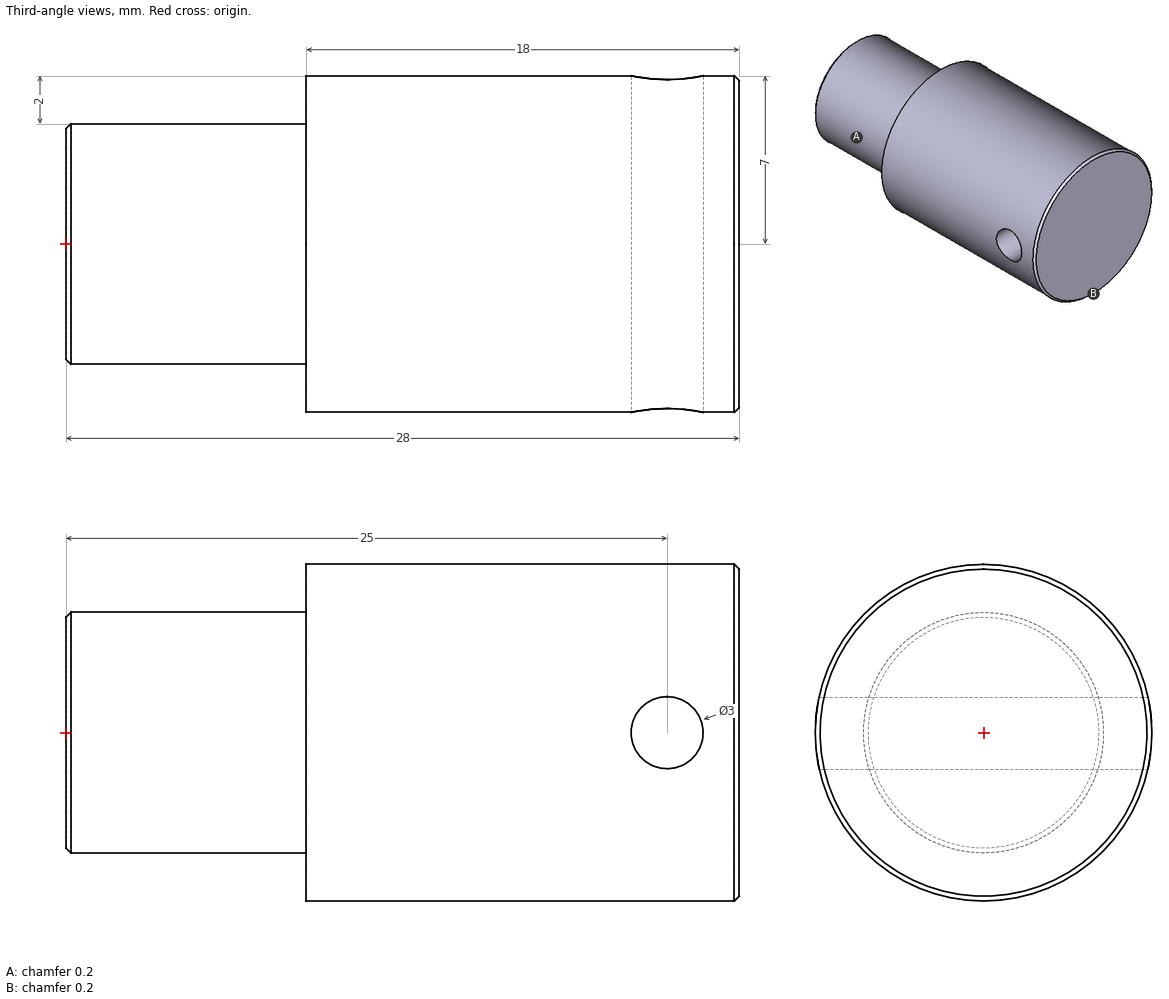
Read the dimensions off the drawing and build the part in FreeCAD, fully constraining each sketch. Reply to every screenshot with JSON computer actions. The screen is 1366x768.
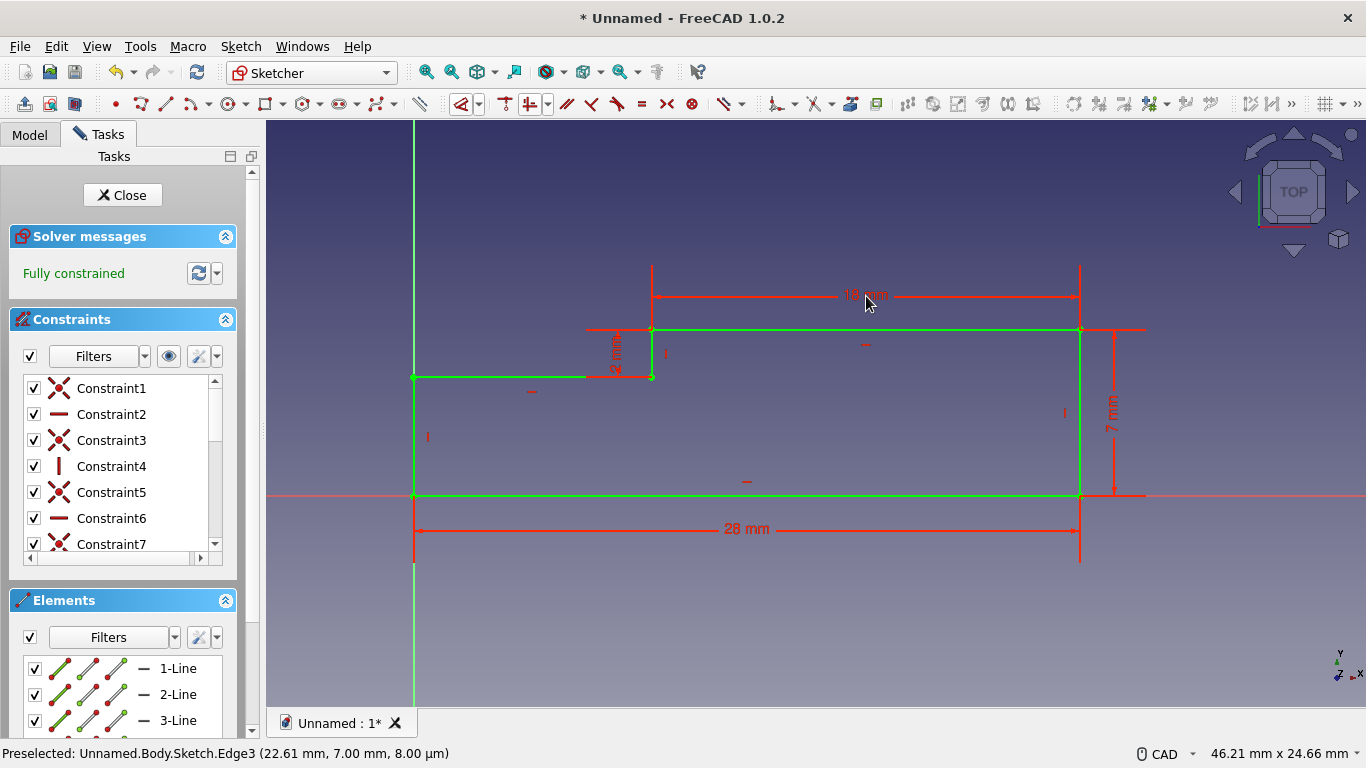
{"action": "left_click", "coordinate": [123, 195]}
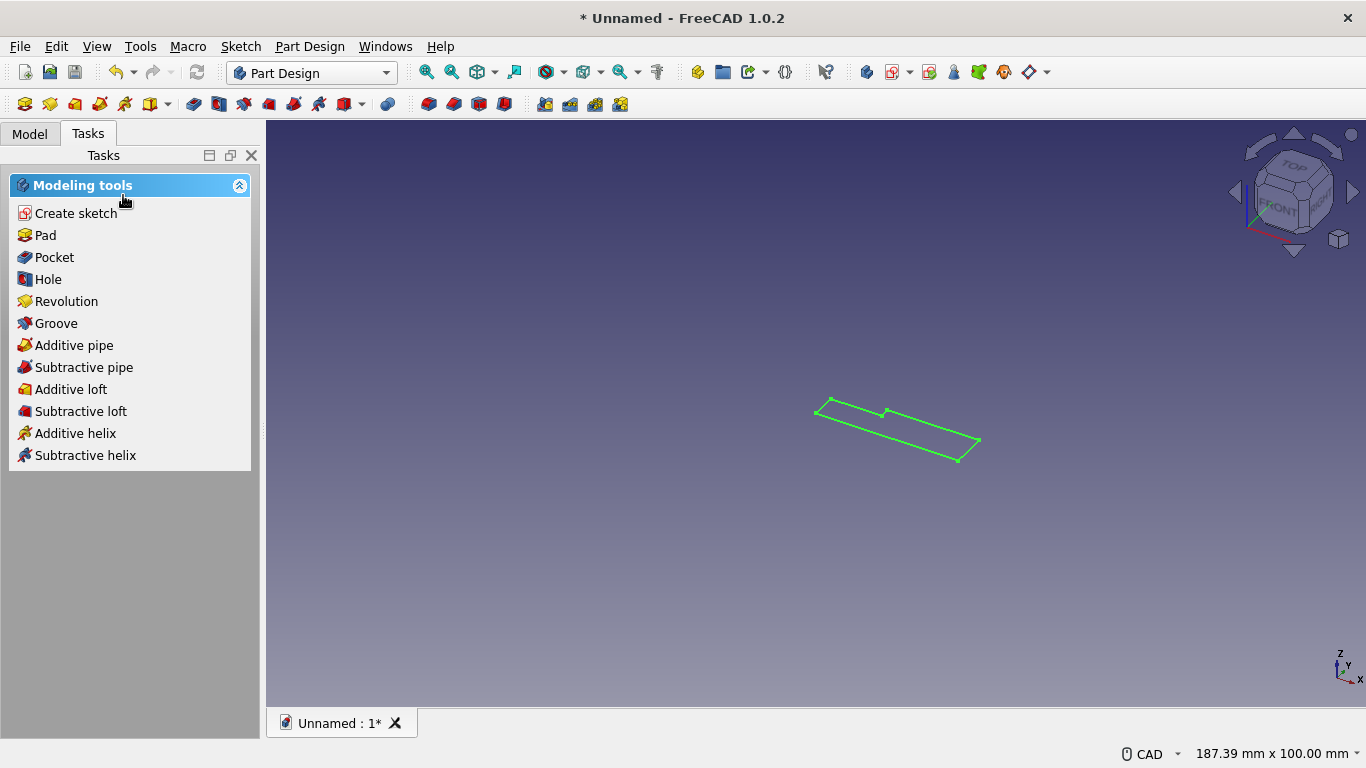
{"action": "left_click", "coordinate": [50, 104]}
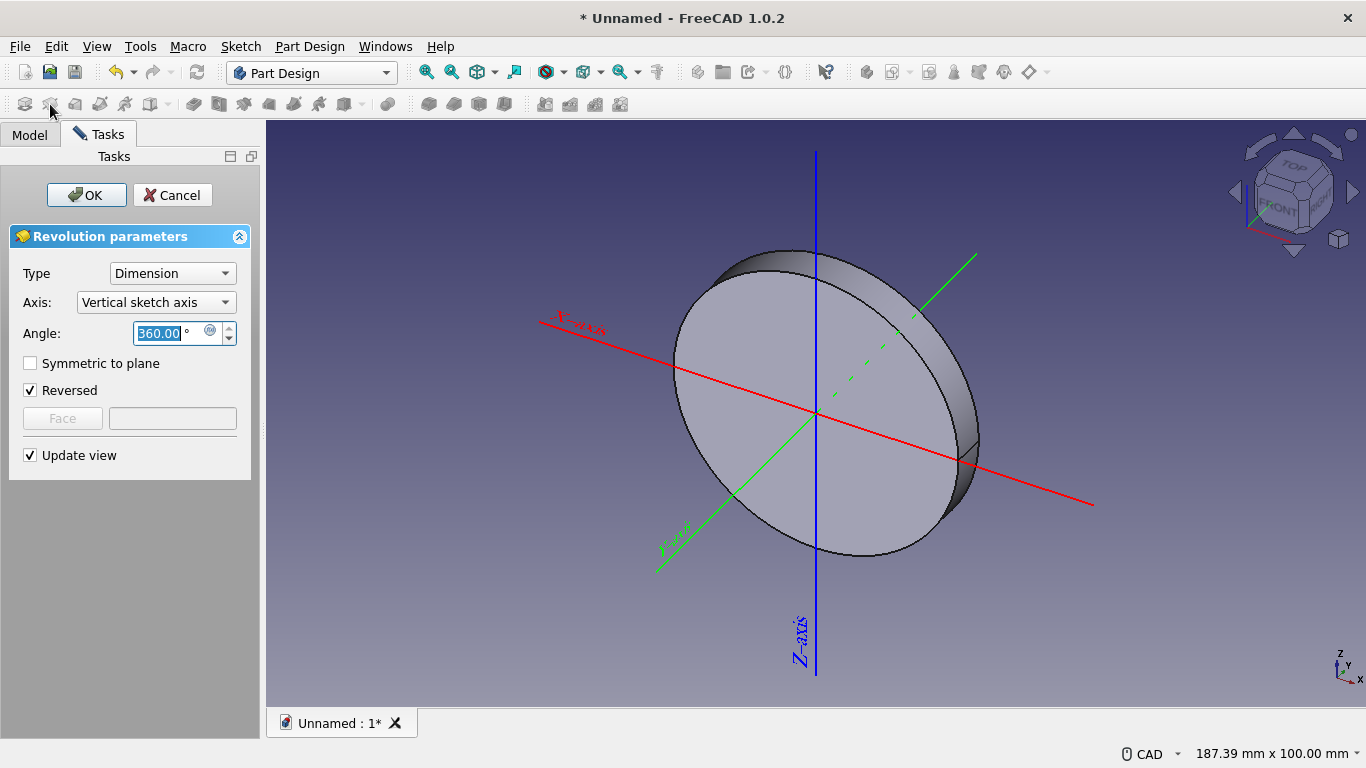
{"action": "left_click", "coordinate": [157, 302]}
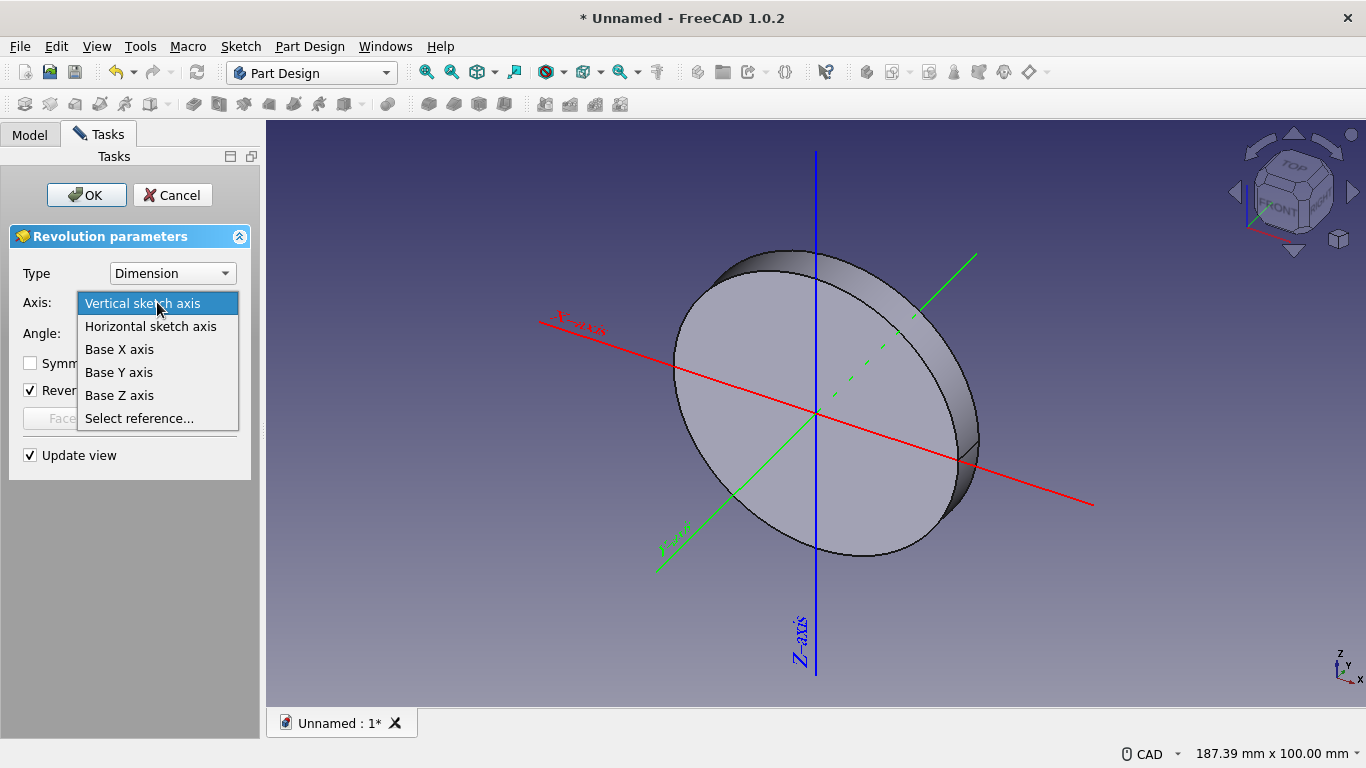
{"action": "left_click", "coordinate": [156, 326]}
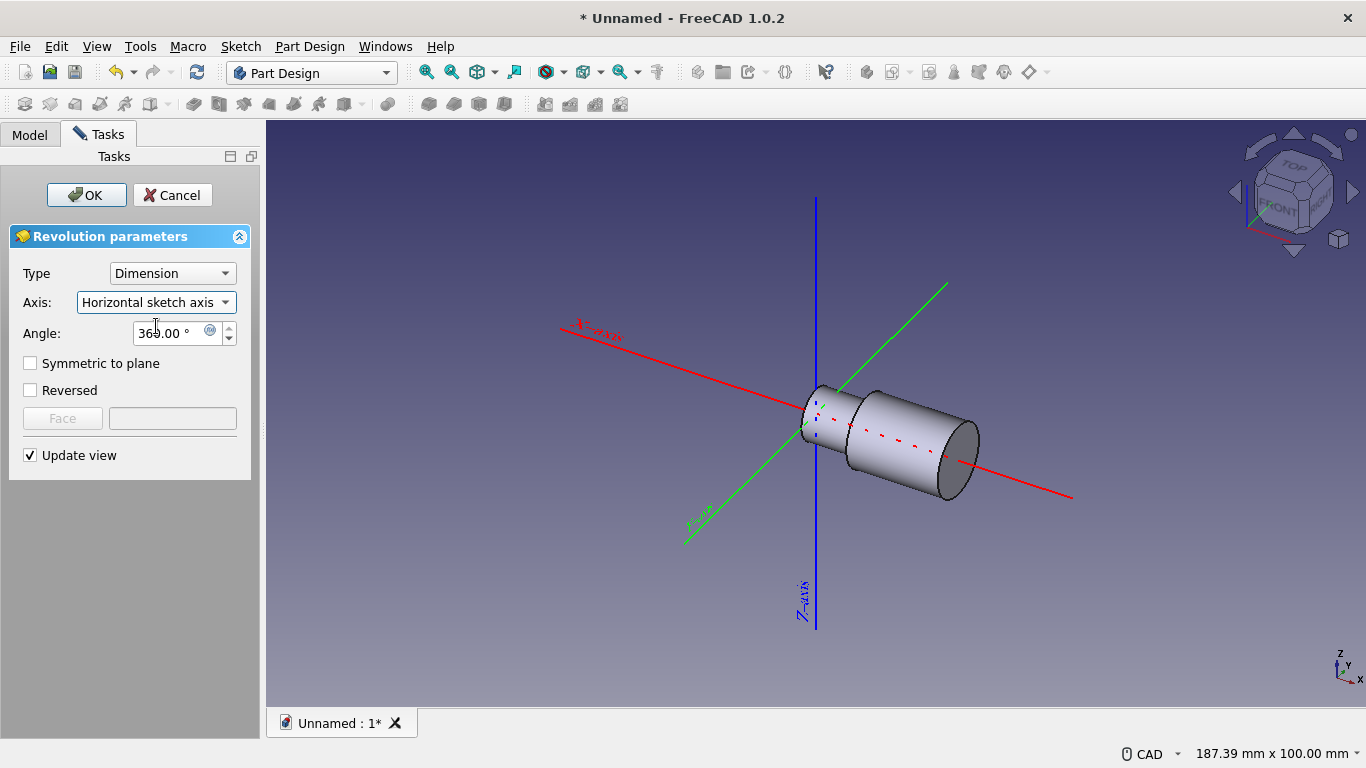
{"action": "left_click", "coordinate": [87, 195]}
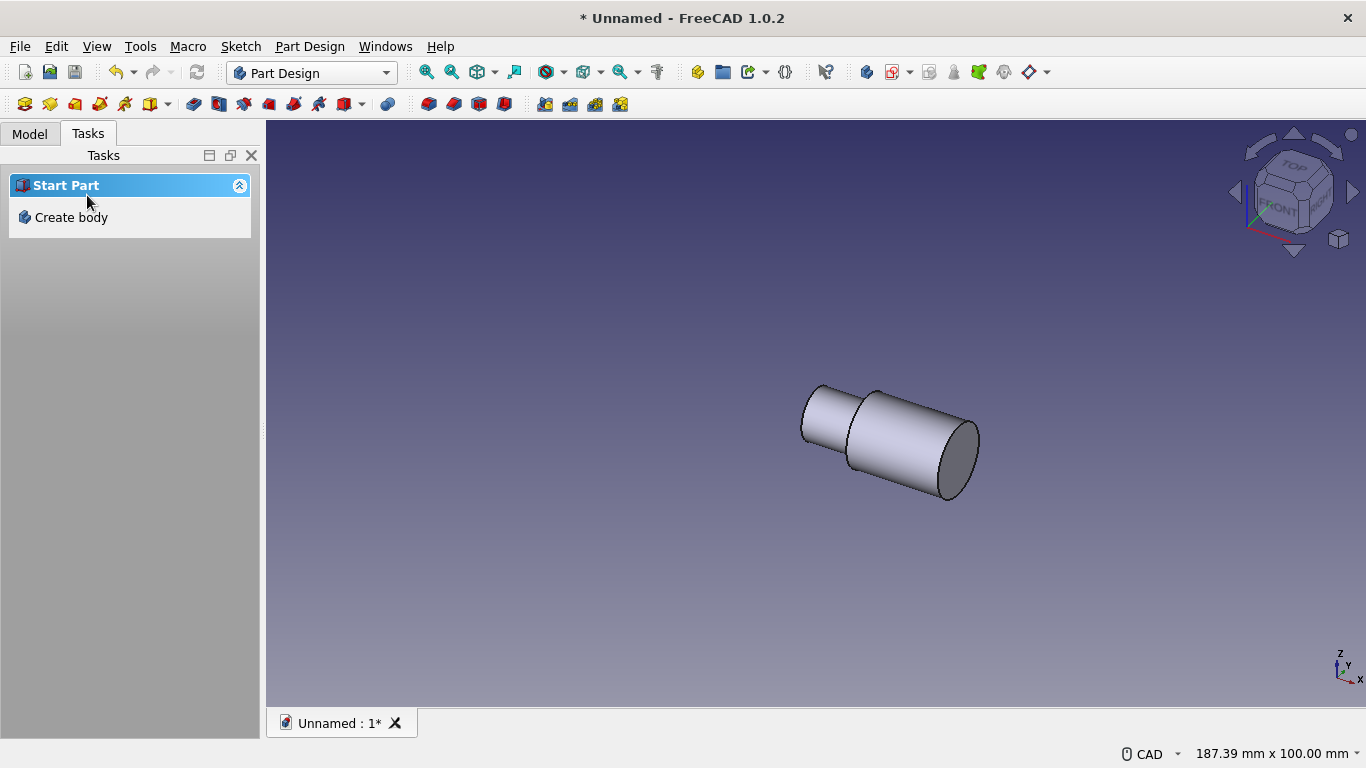
{"action": "left_click", "coordinate": [427, 72]}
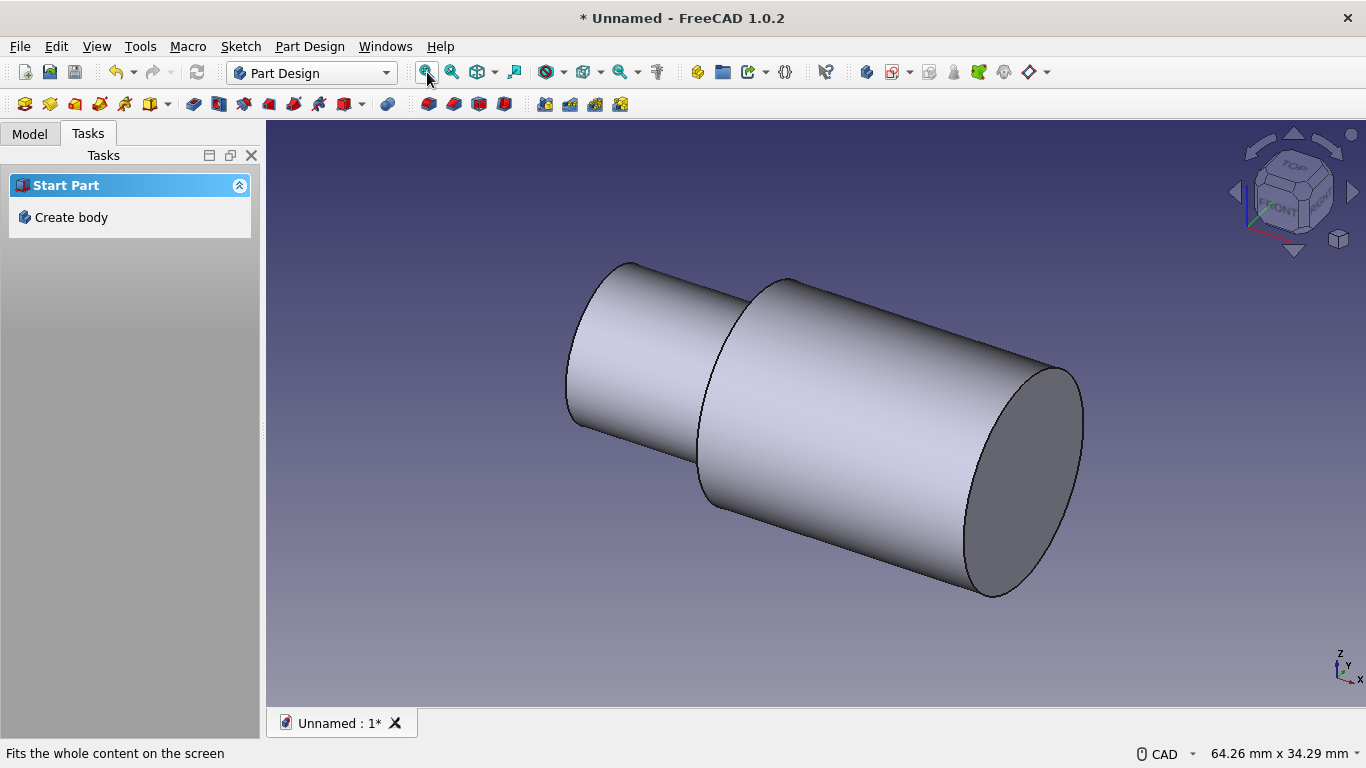
{"action": "key", "text": "0"}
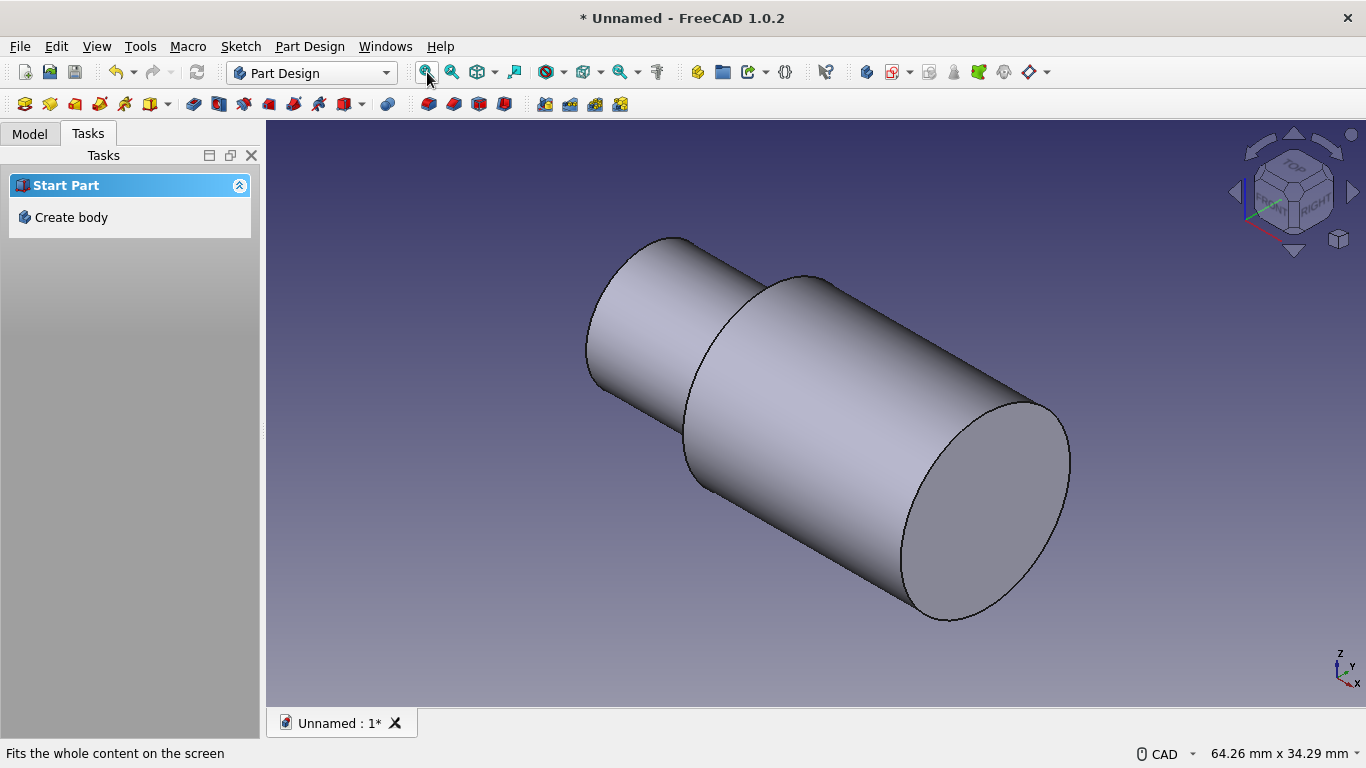
{"action": "key", "text": "2"}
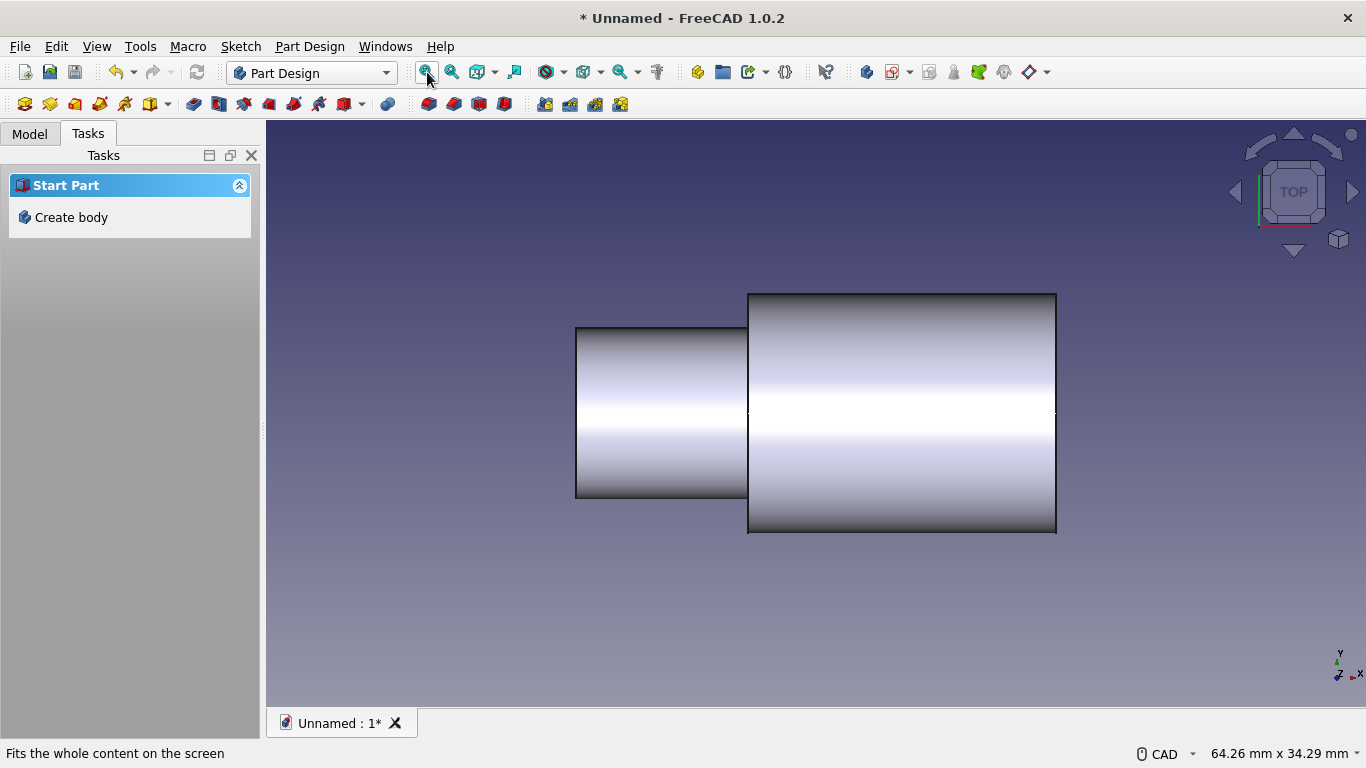
{"action": "left_click", "coordinate": [427, 72]}